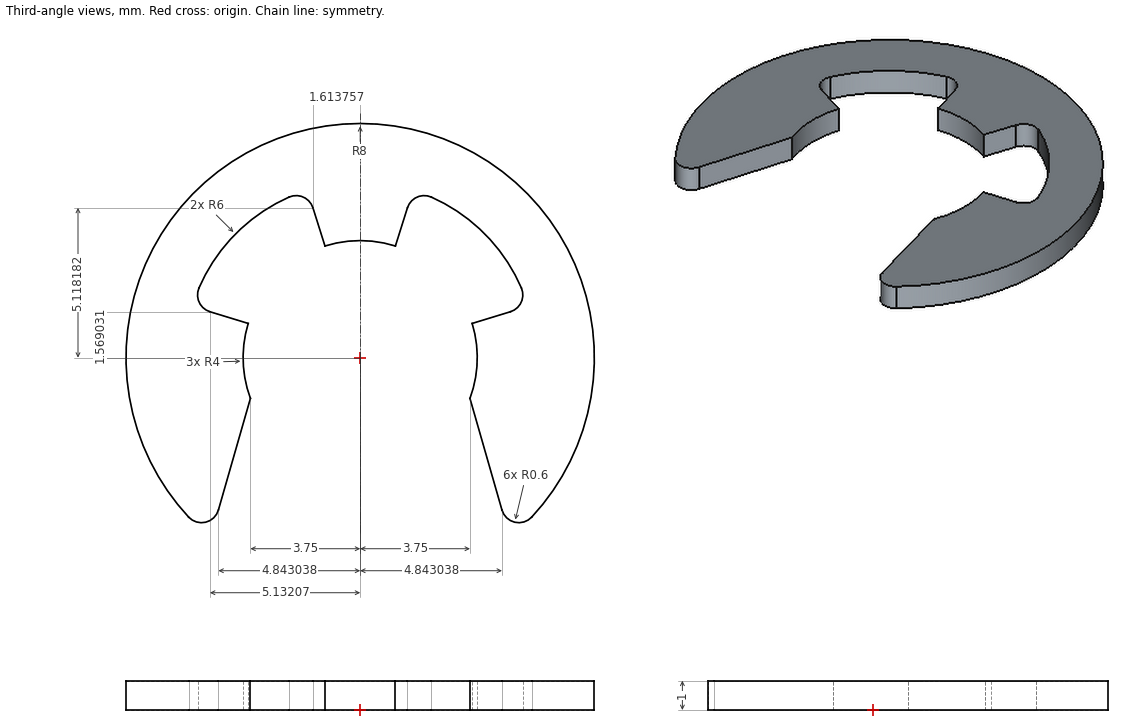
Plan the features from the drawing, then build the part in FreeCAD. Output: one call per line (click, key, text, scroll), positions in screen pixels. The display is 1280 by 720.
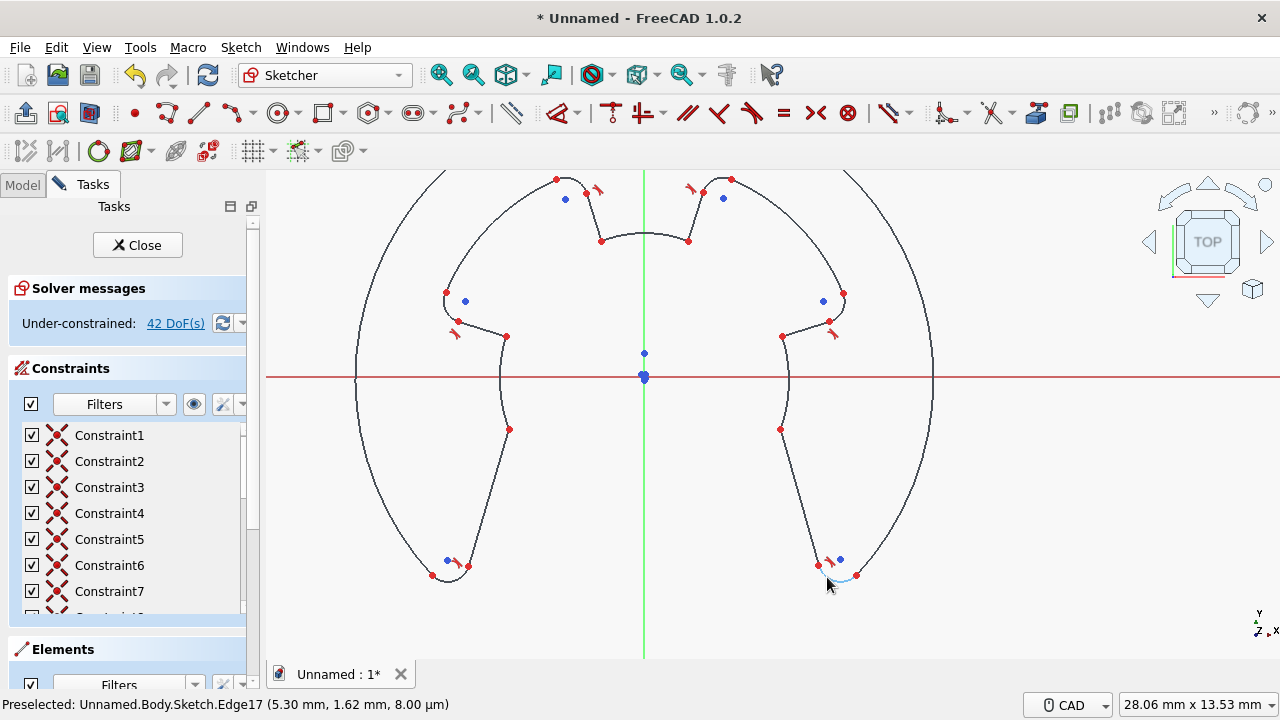
click(827, 577)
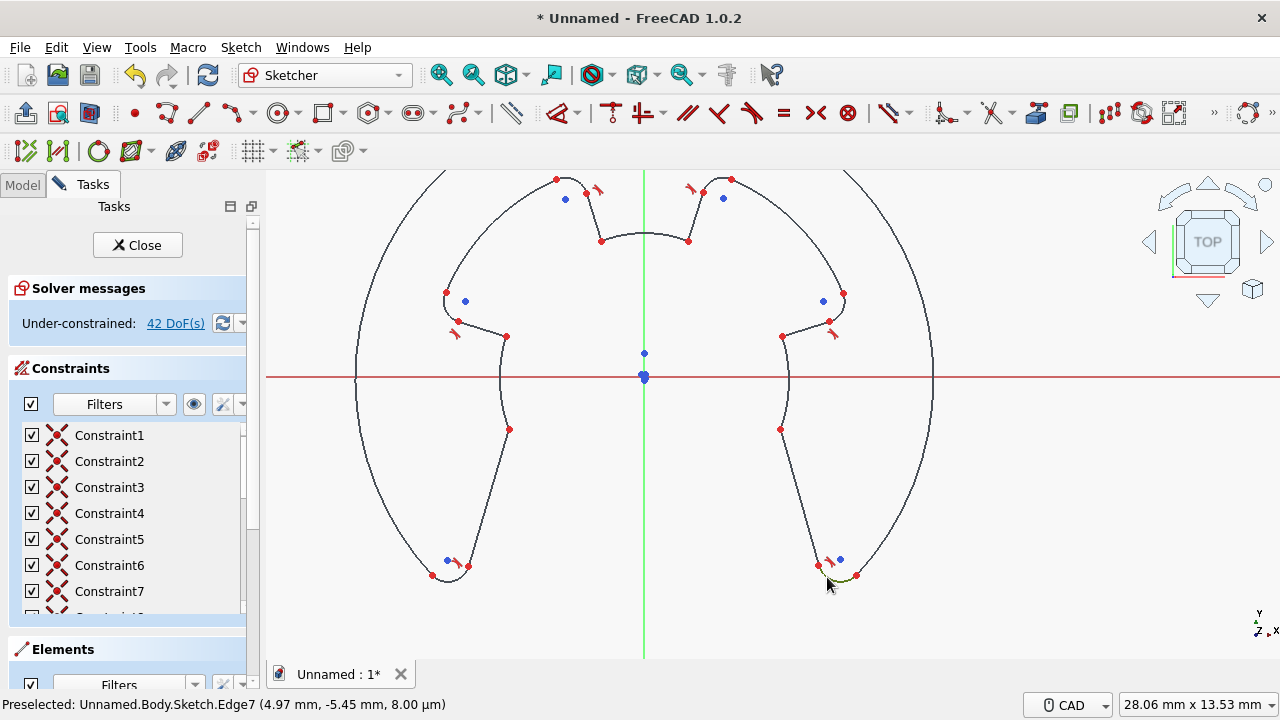
click(876, 205)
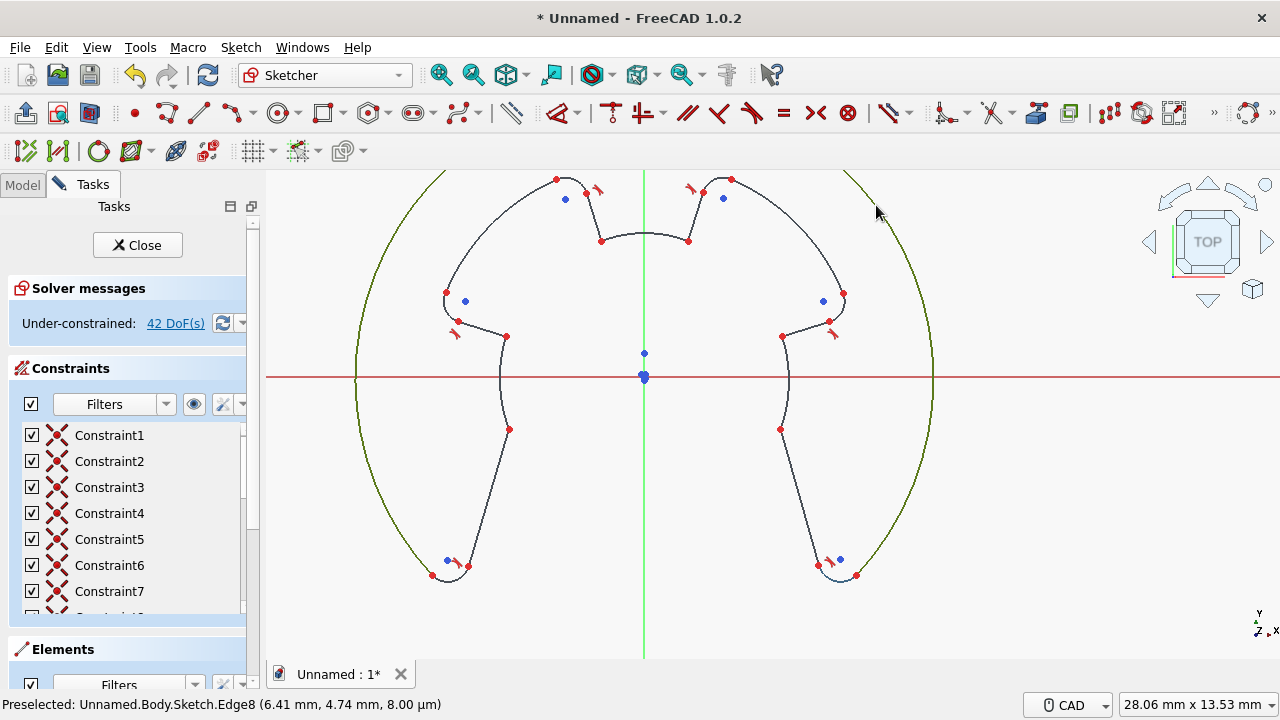
click(752, 114)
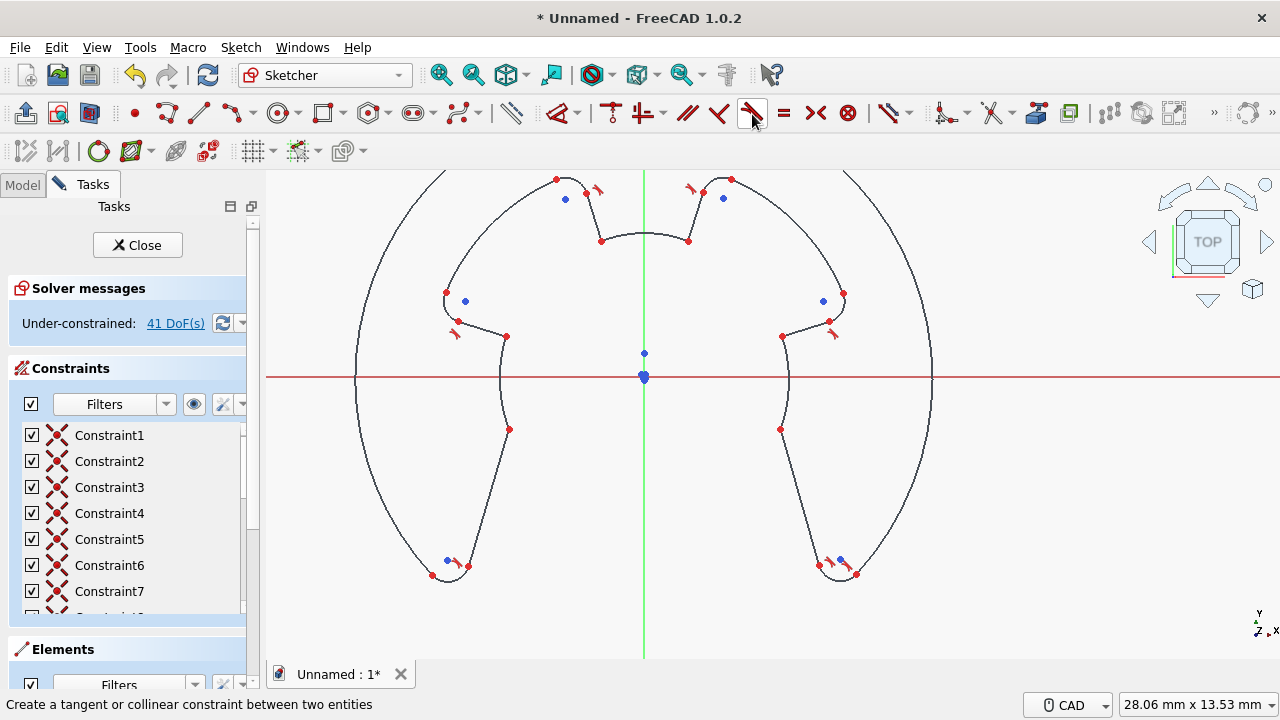
click(874, 205)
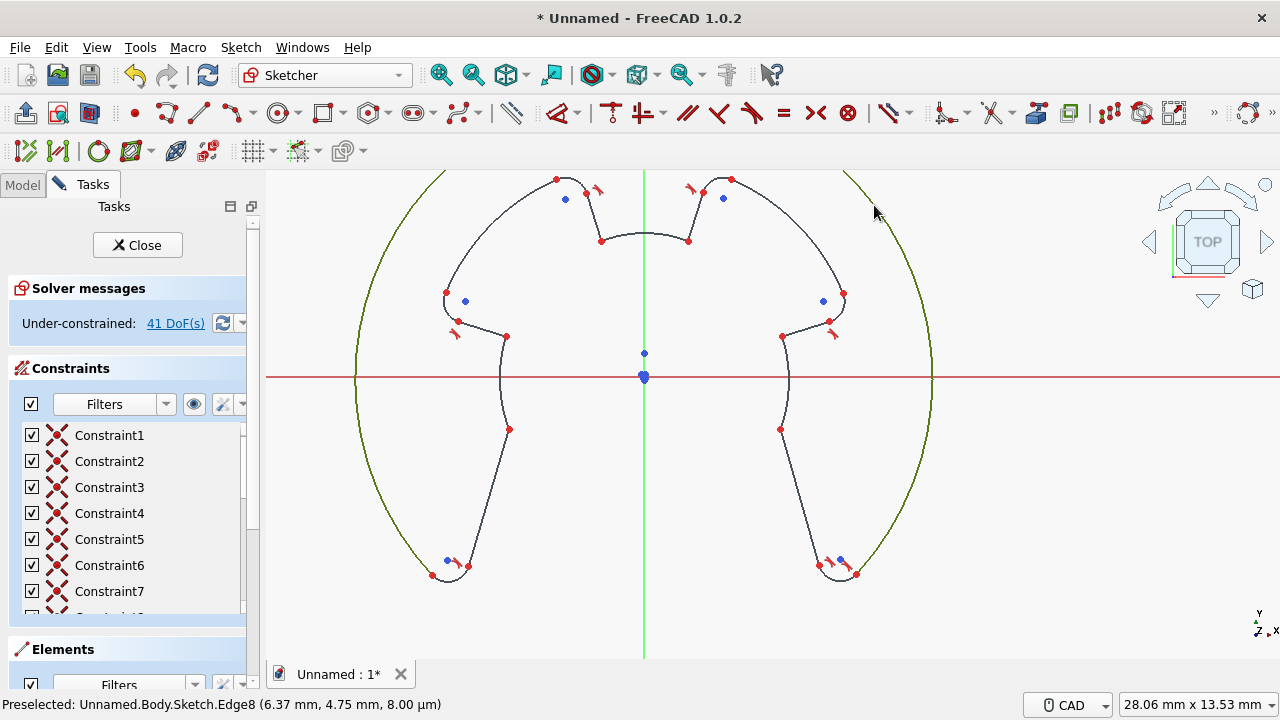
click(445, 582)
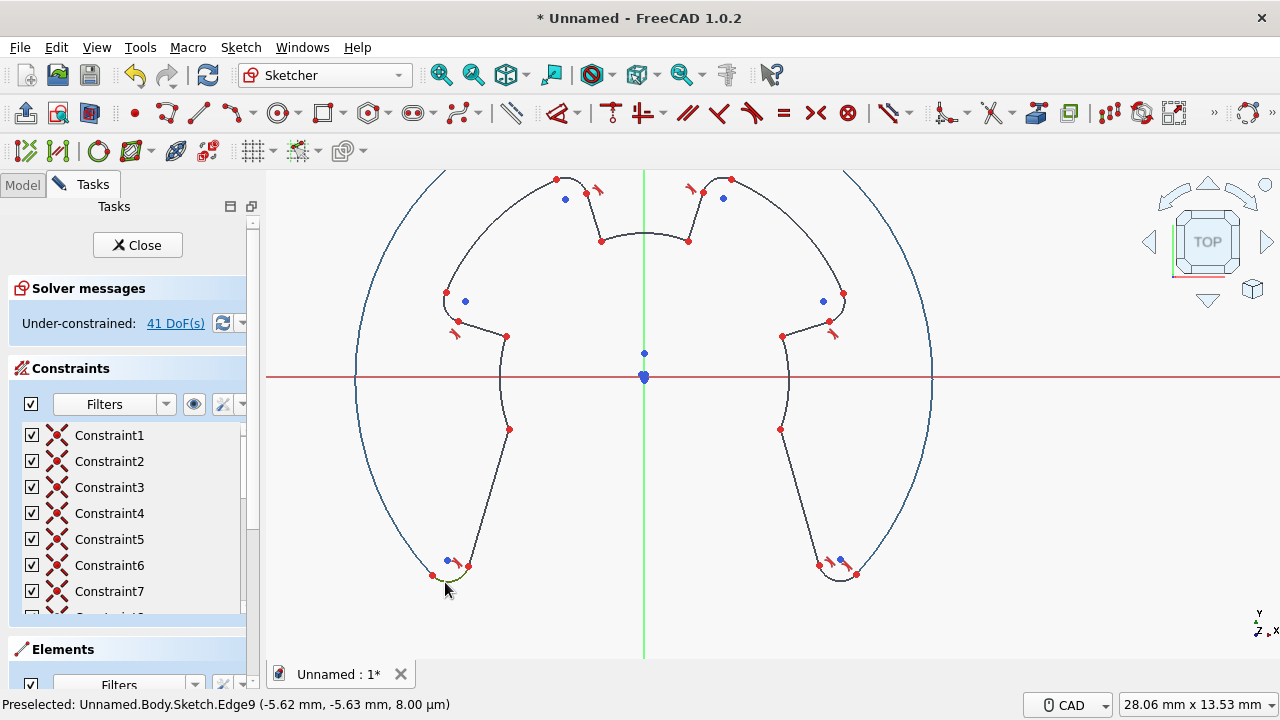
click(752, 114)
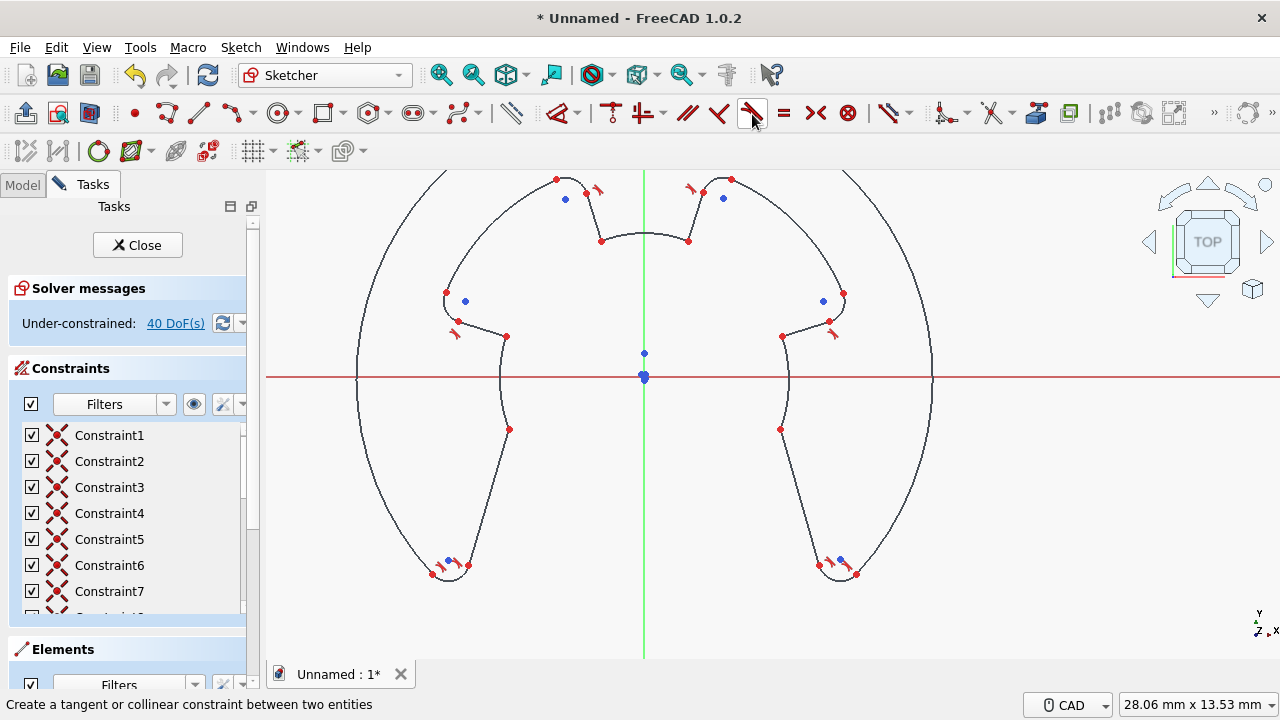
scroll(444, 303, up, 2)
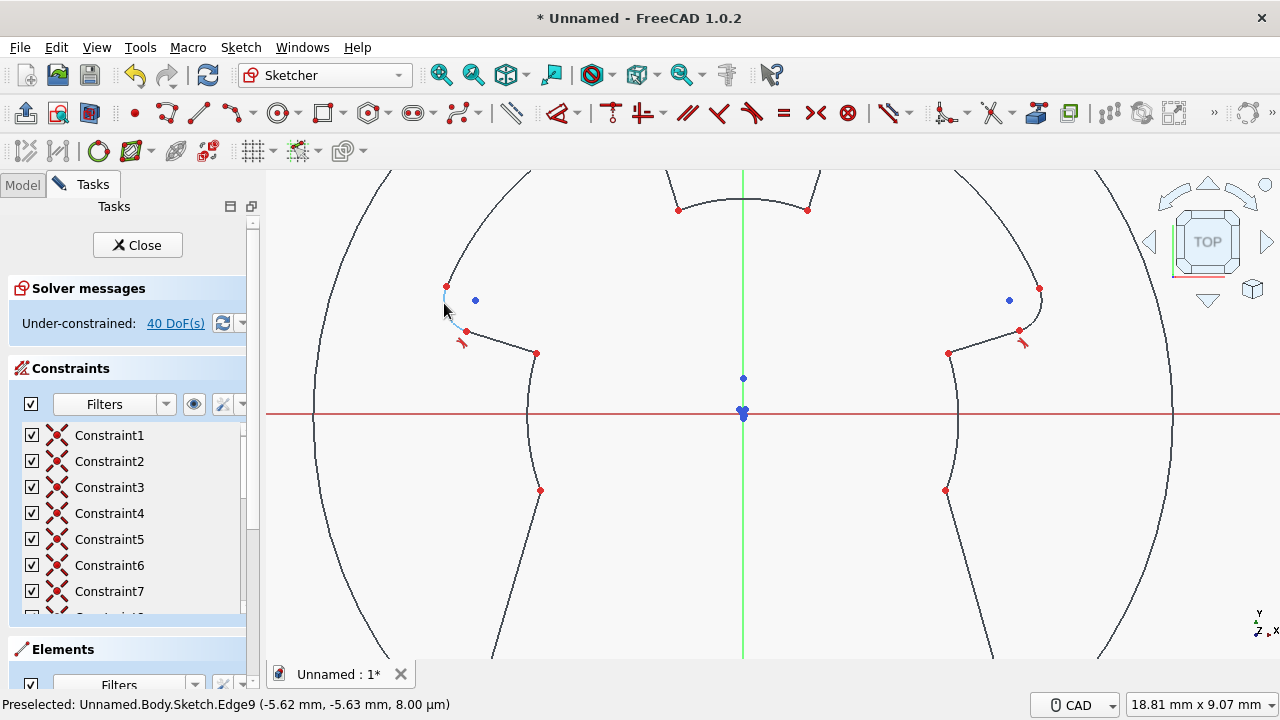
click(444, 303)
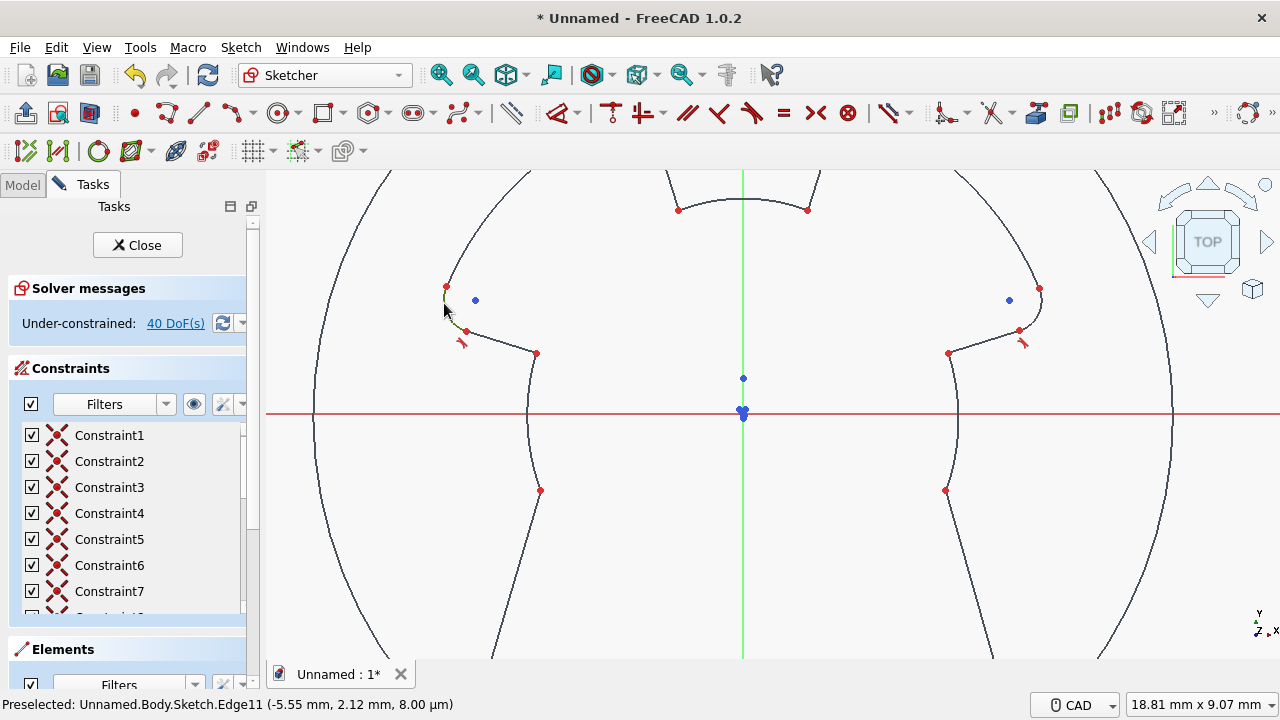
click(482, 224)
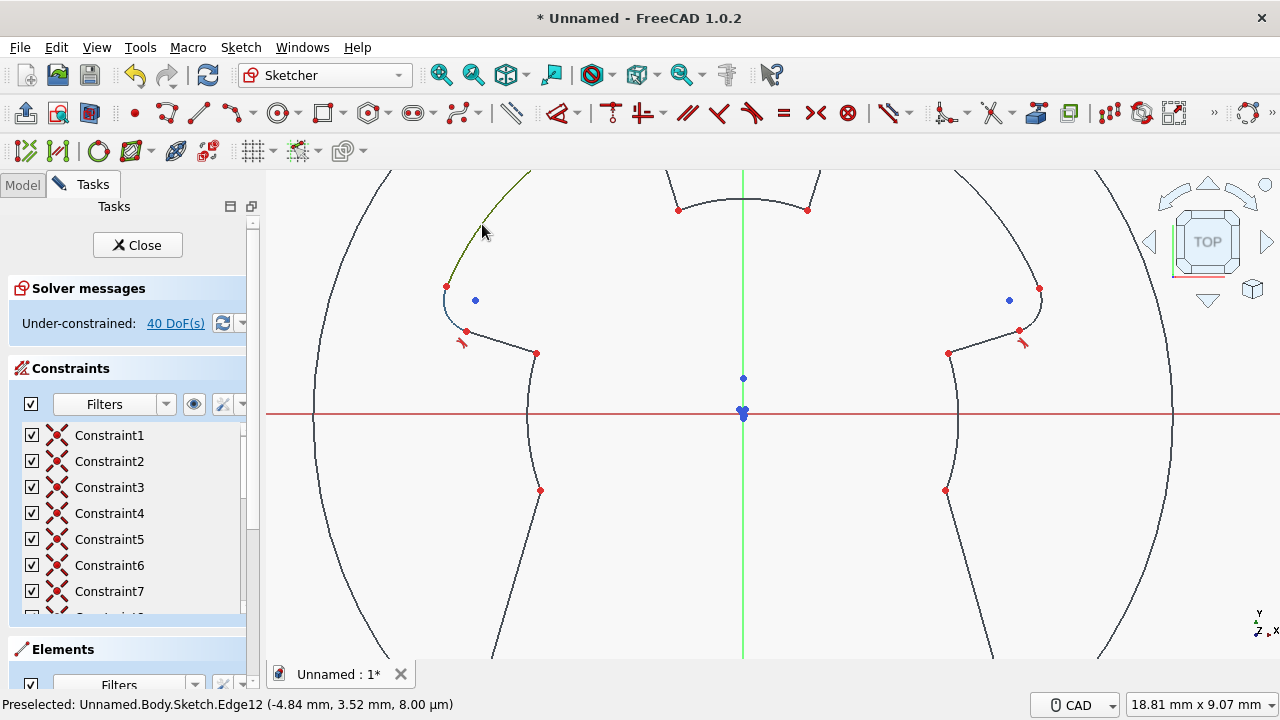
key(t)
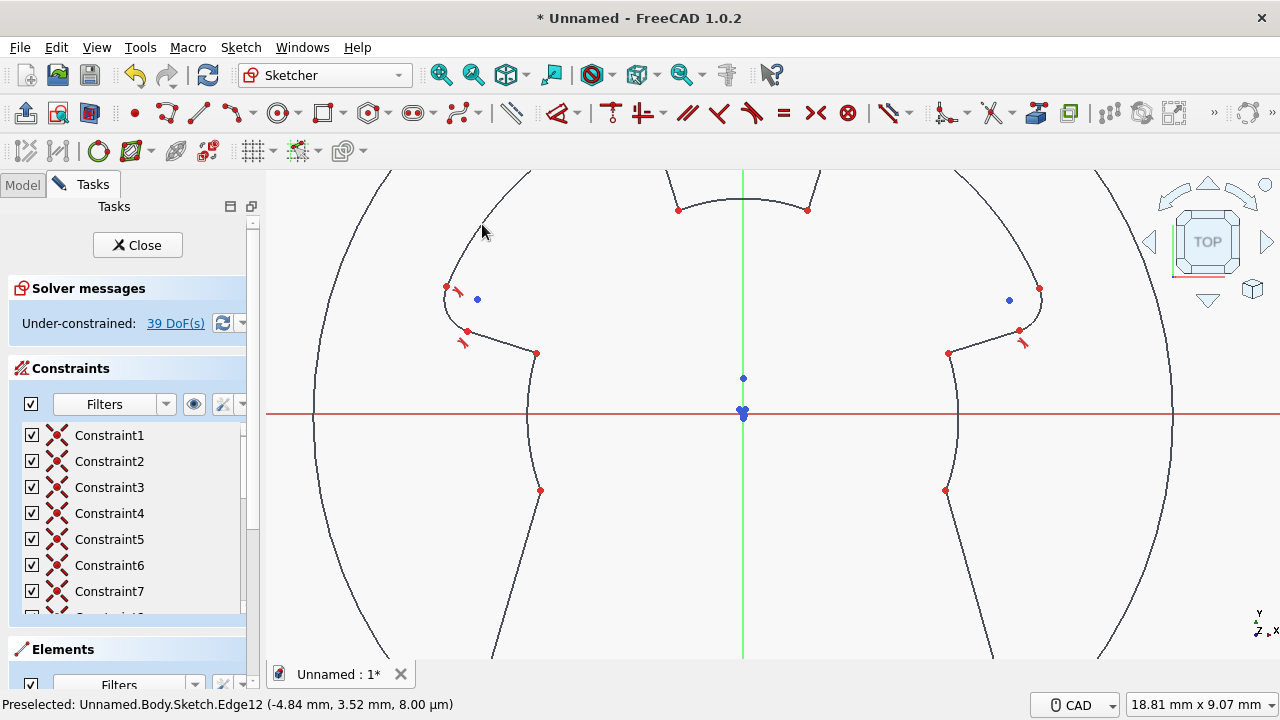
click(482, 224)